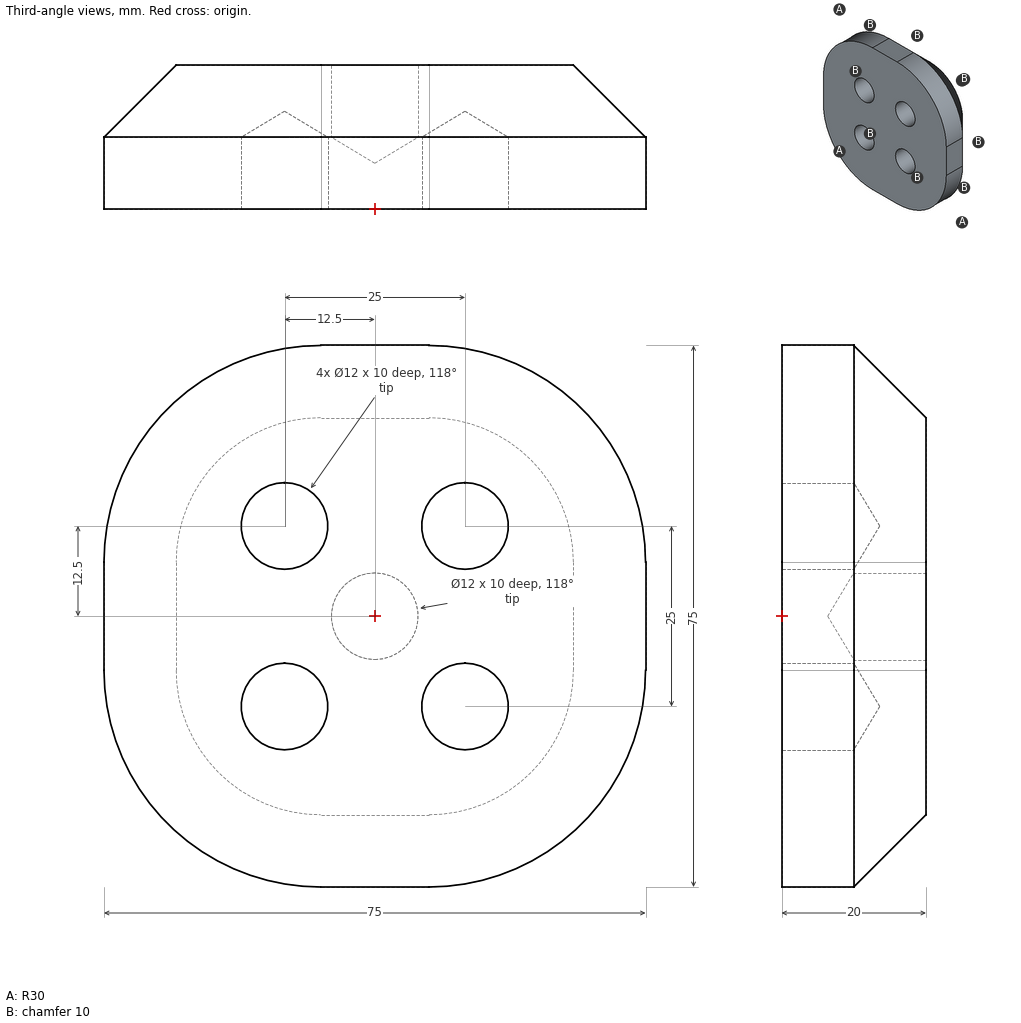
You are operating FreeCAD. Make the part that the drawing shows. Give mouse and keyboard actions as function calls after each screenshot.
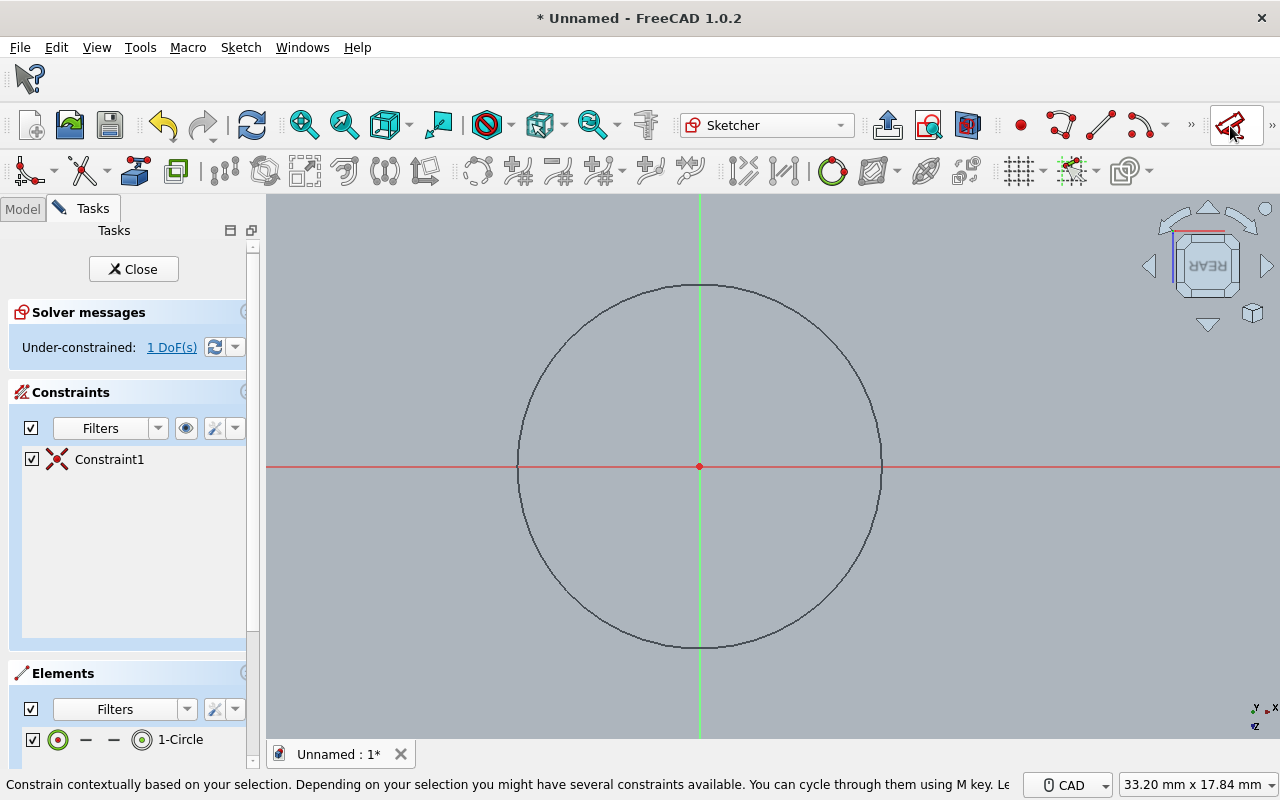
click(828, 337)
click(851, 314)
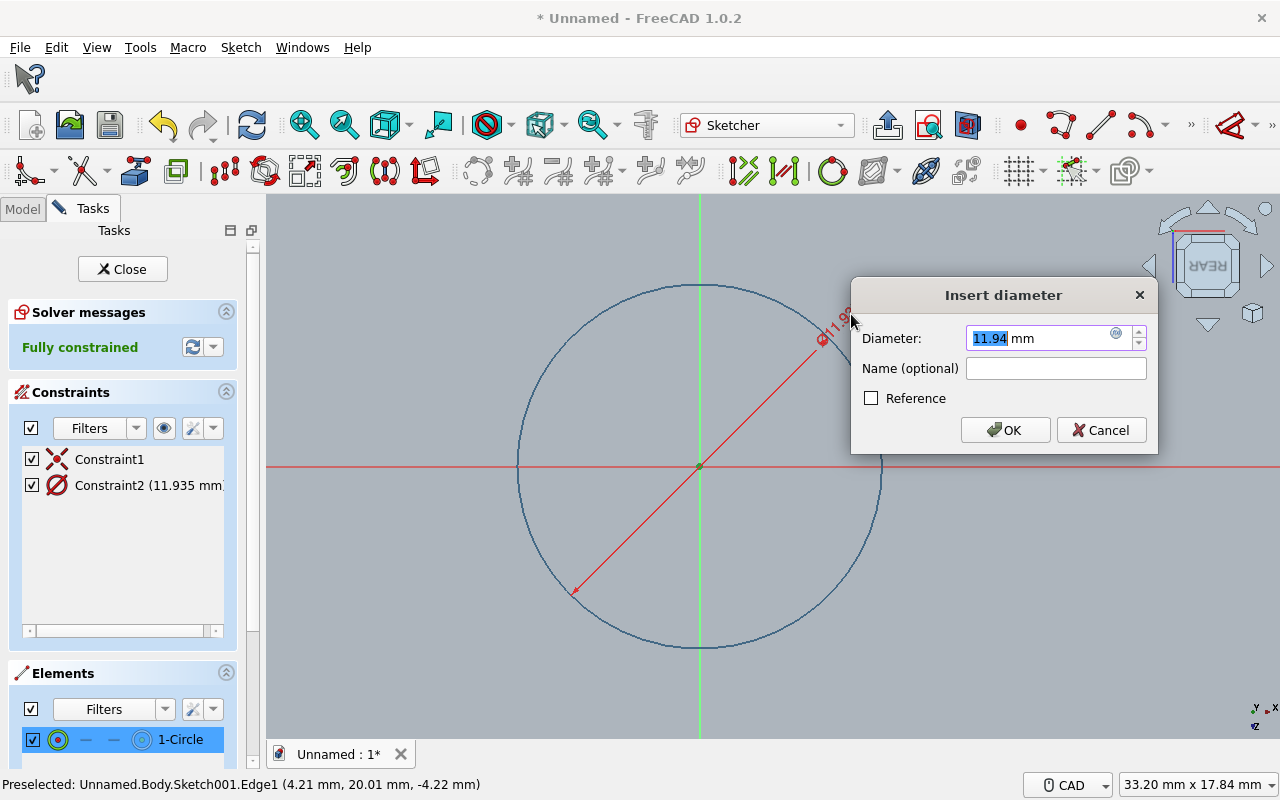
text(12)
key(Return)
key(Escape)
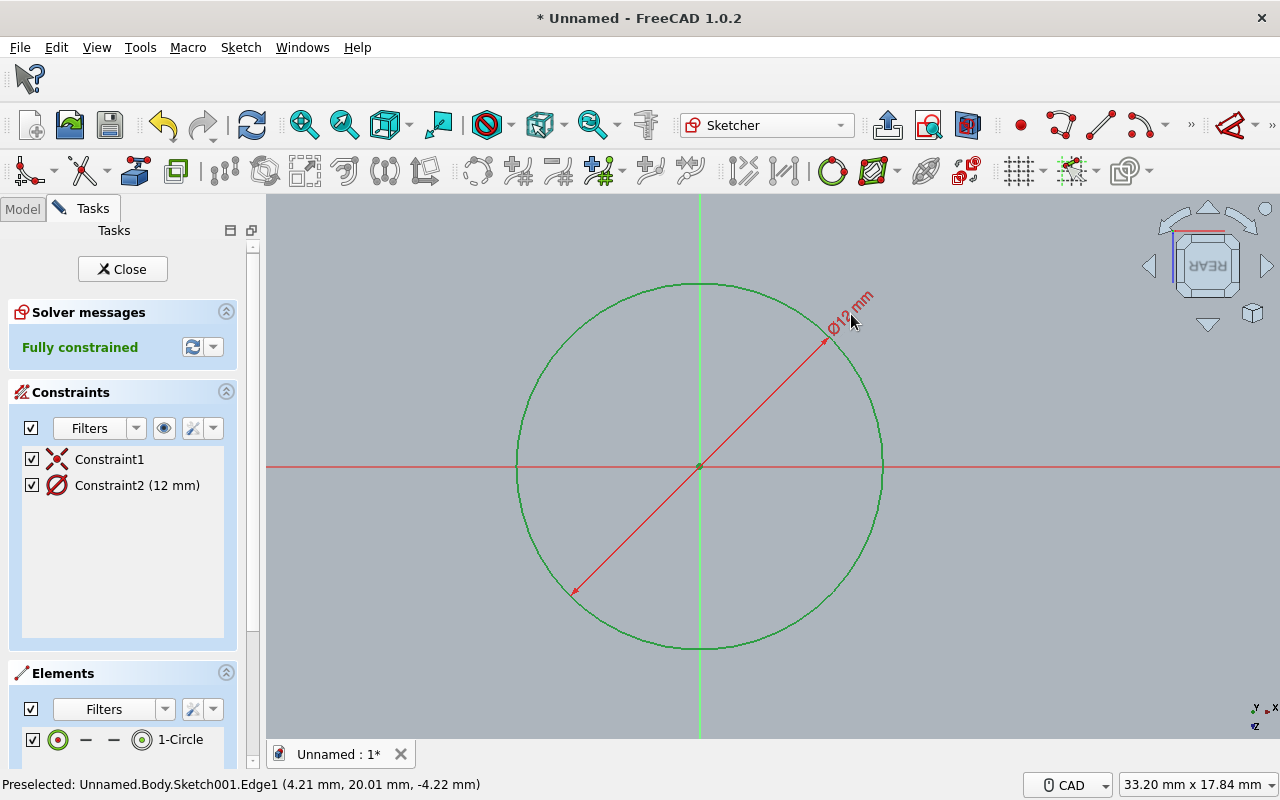
click(123, 269)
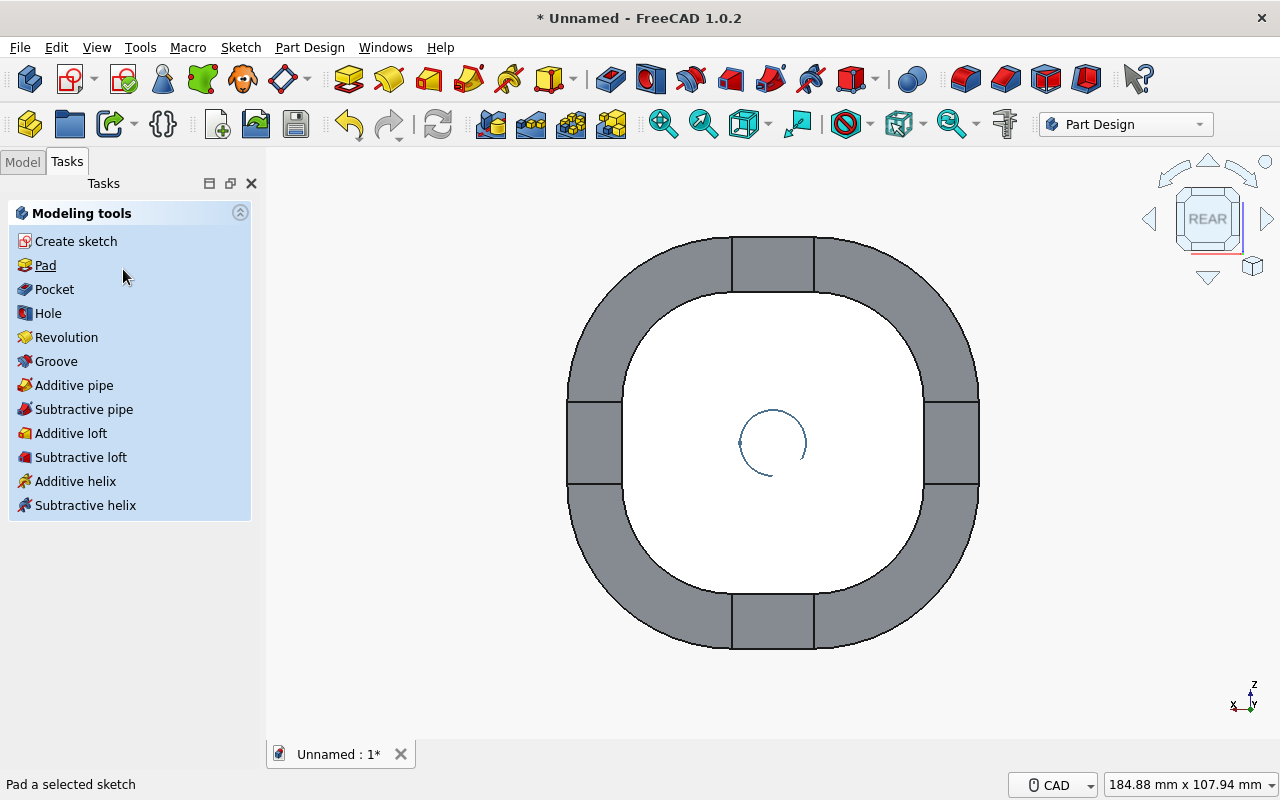
click(652, 80)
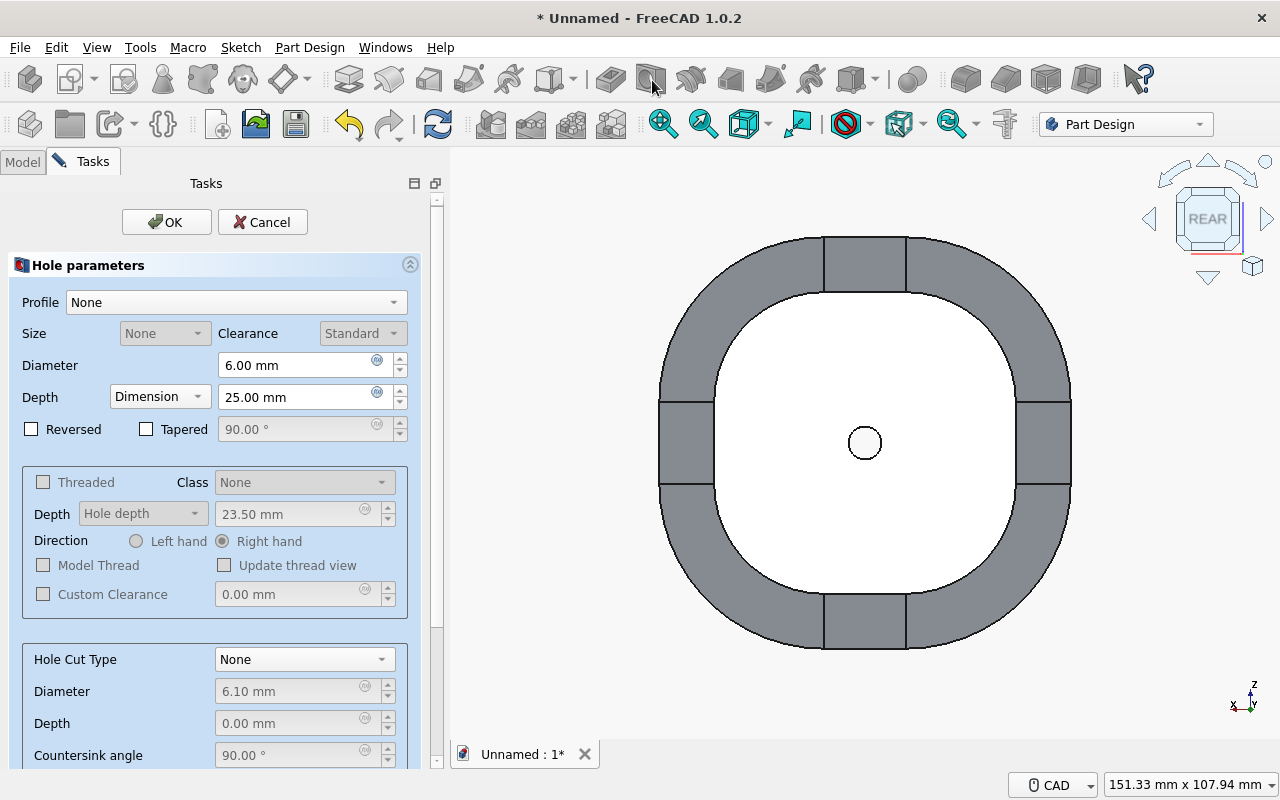
triple_click(305, 365)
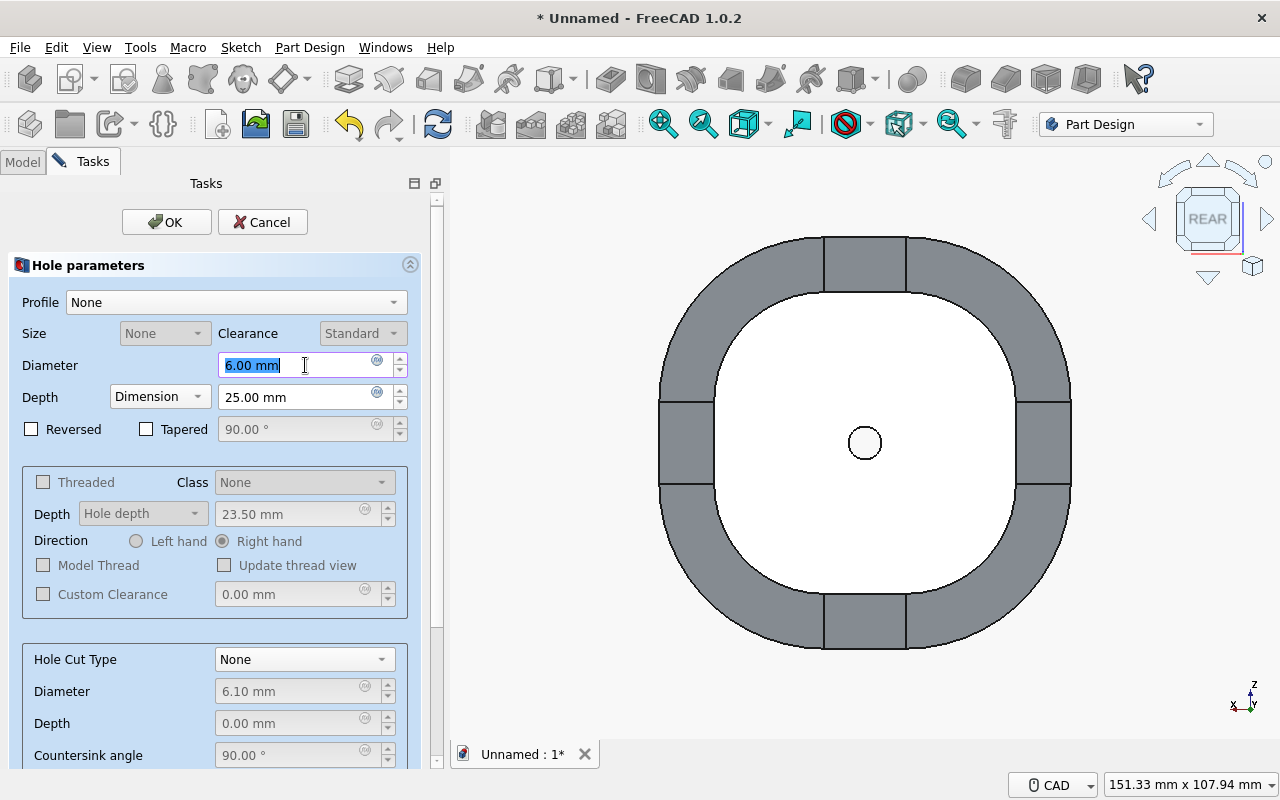
text(12)
key(Tab)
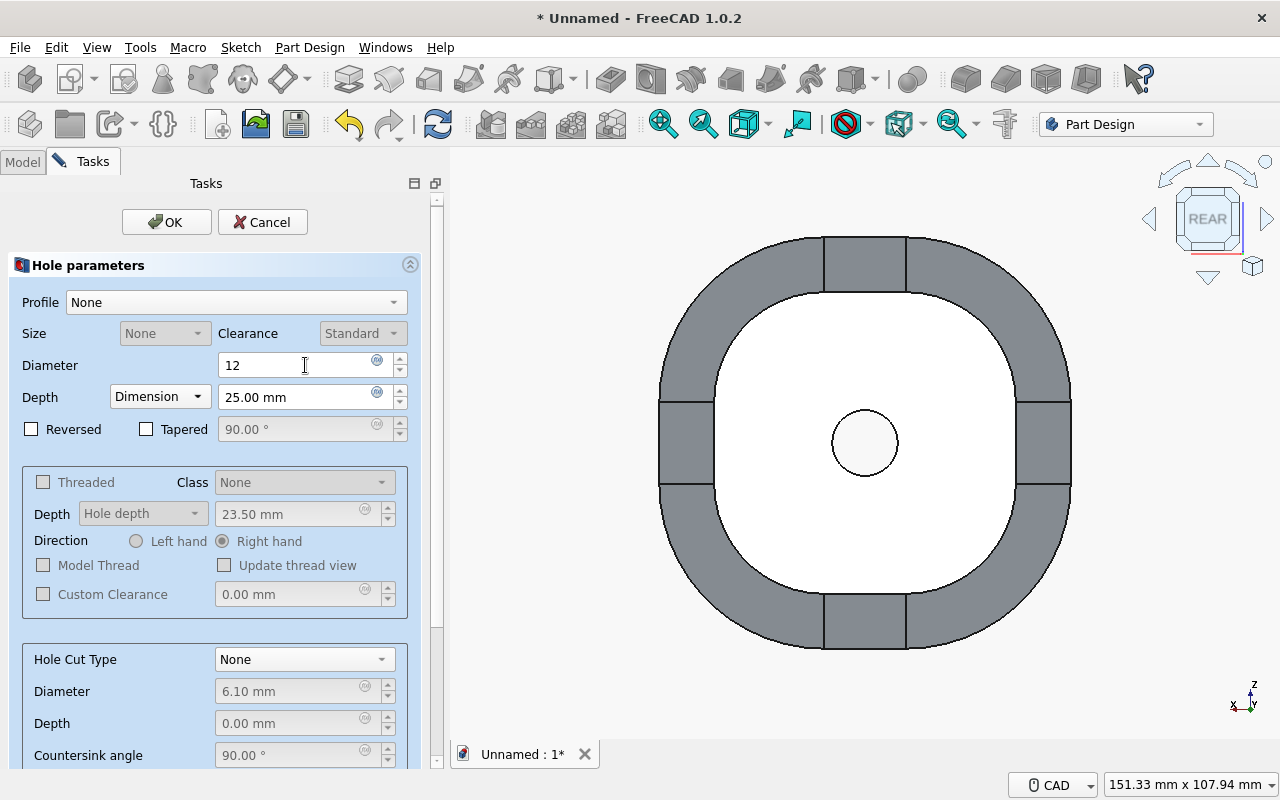
triple_click(305, 397)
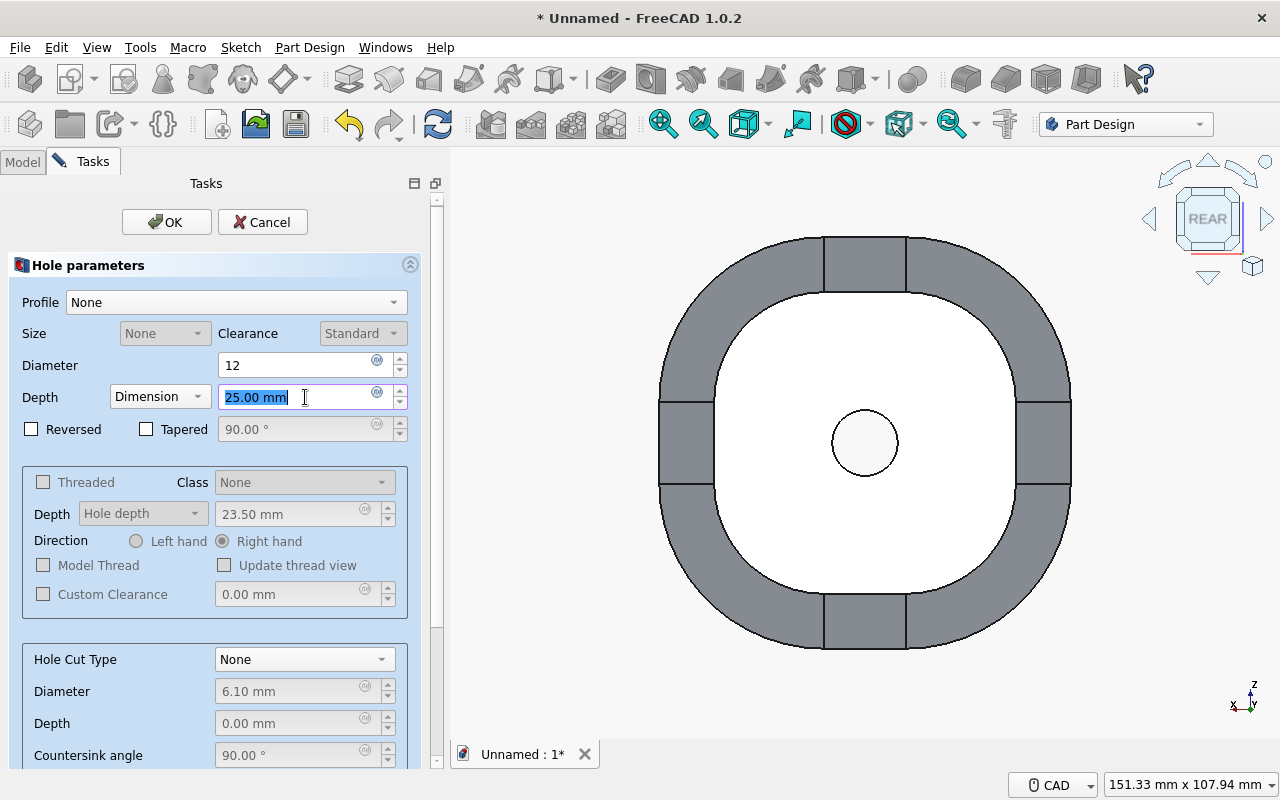
text(10)
key(Tab)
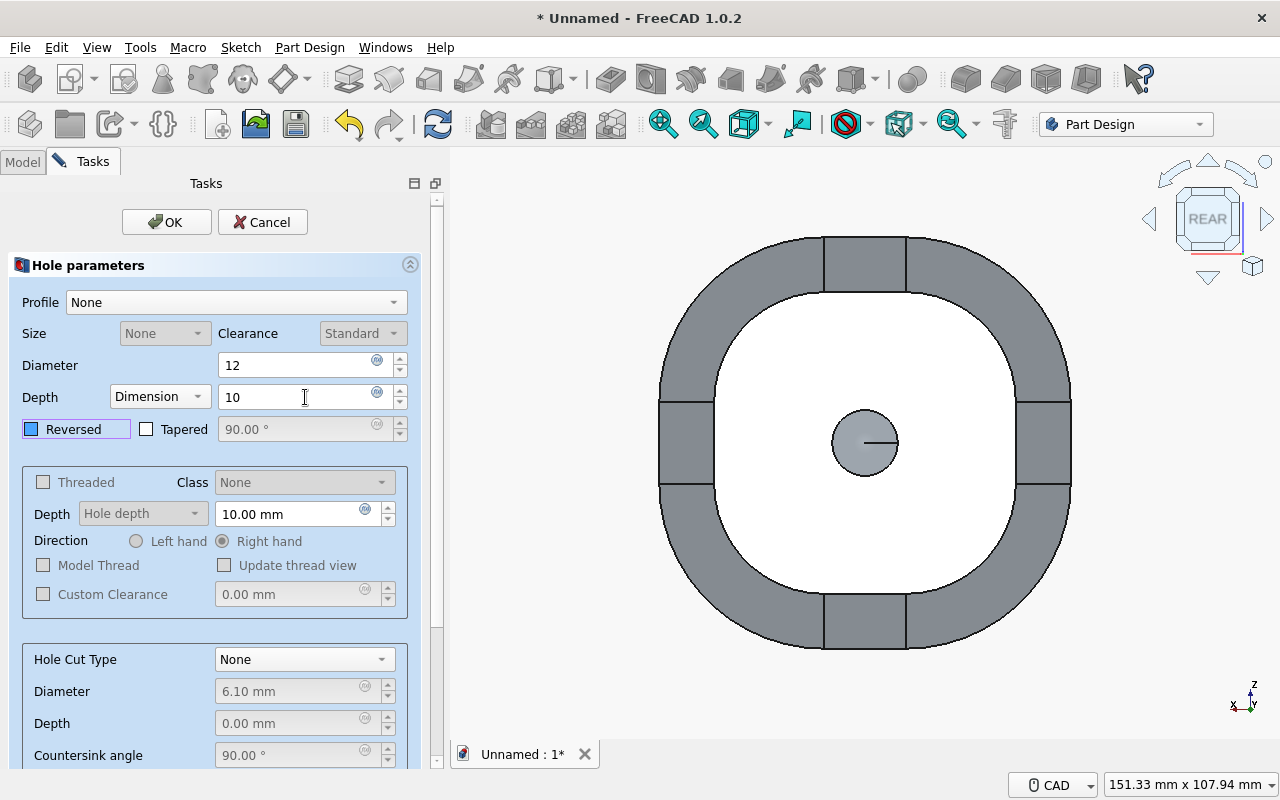
click(167, 222)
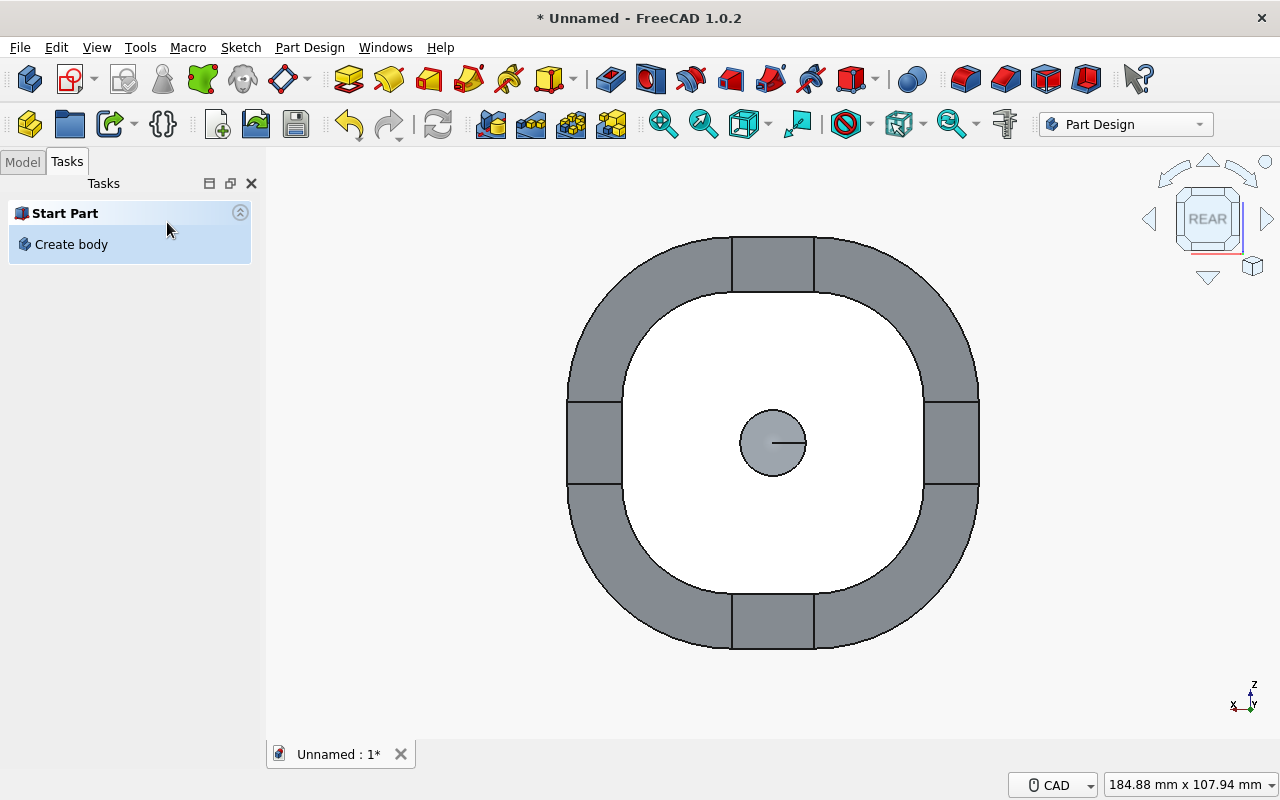
key(0)